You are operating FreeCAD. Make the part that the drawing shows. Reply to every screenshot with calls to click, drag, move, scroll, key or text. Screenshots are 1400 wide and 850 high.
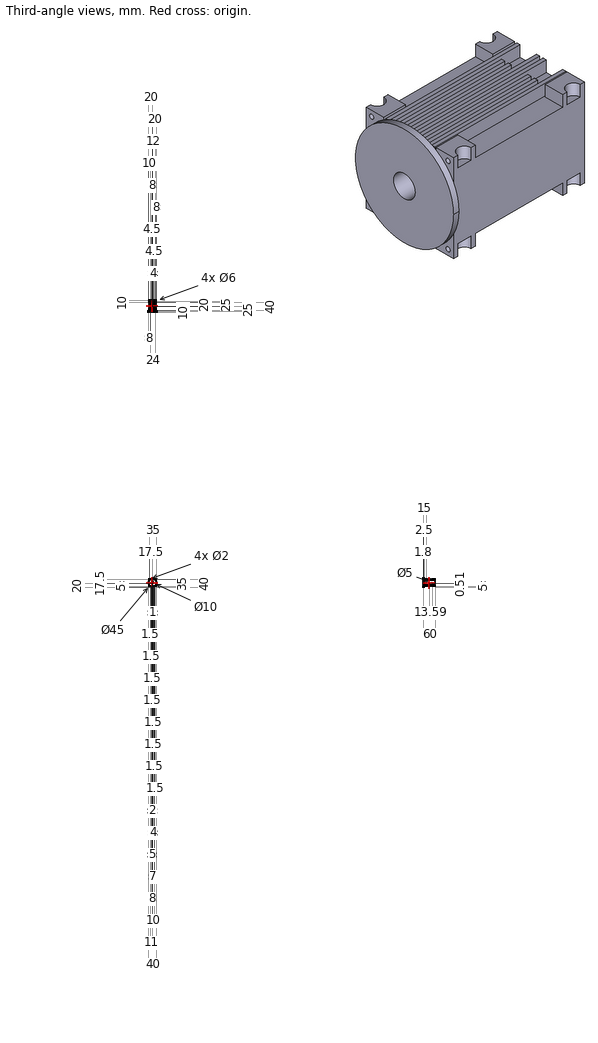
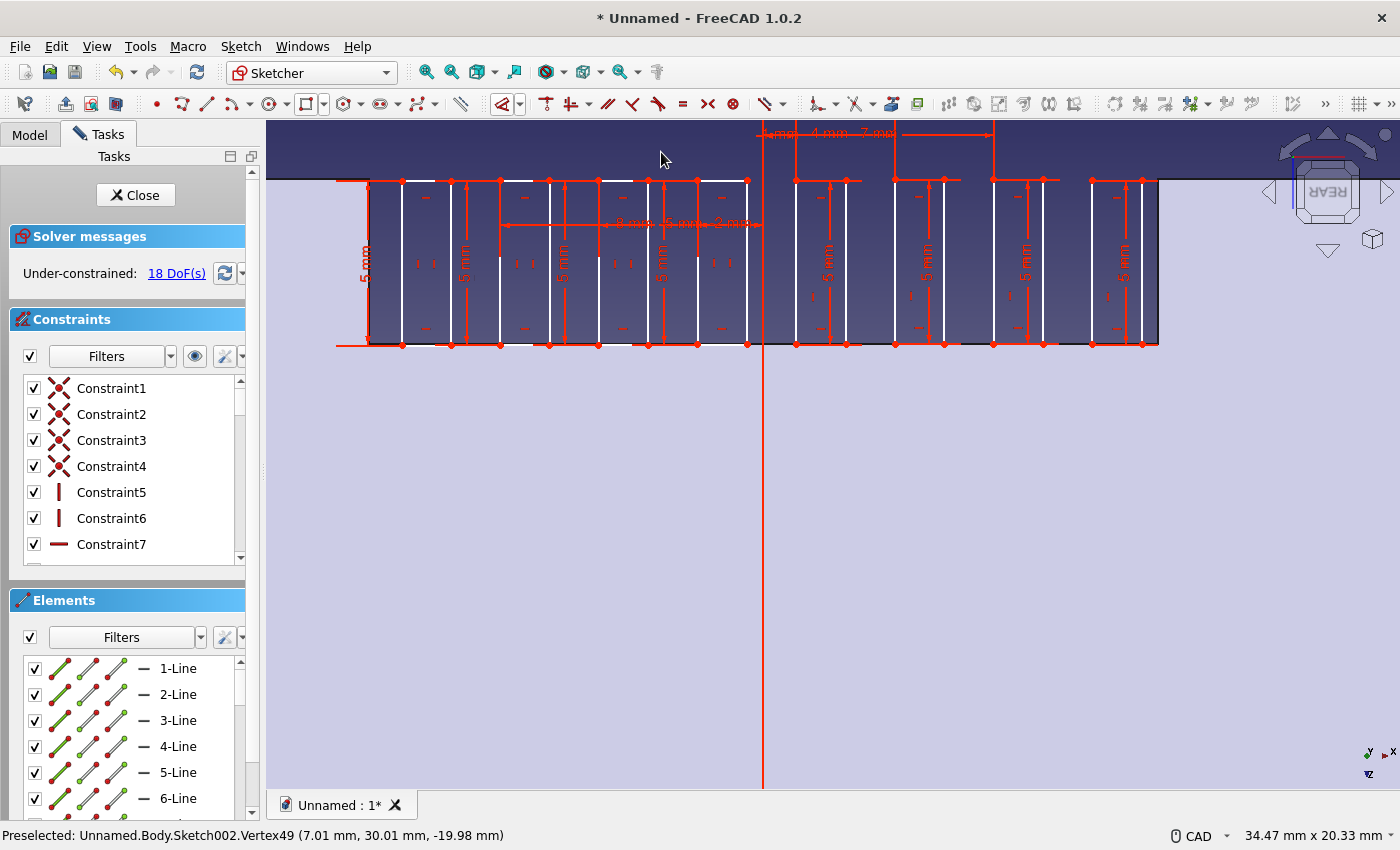
click(417, 346)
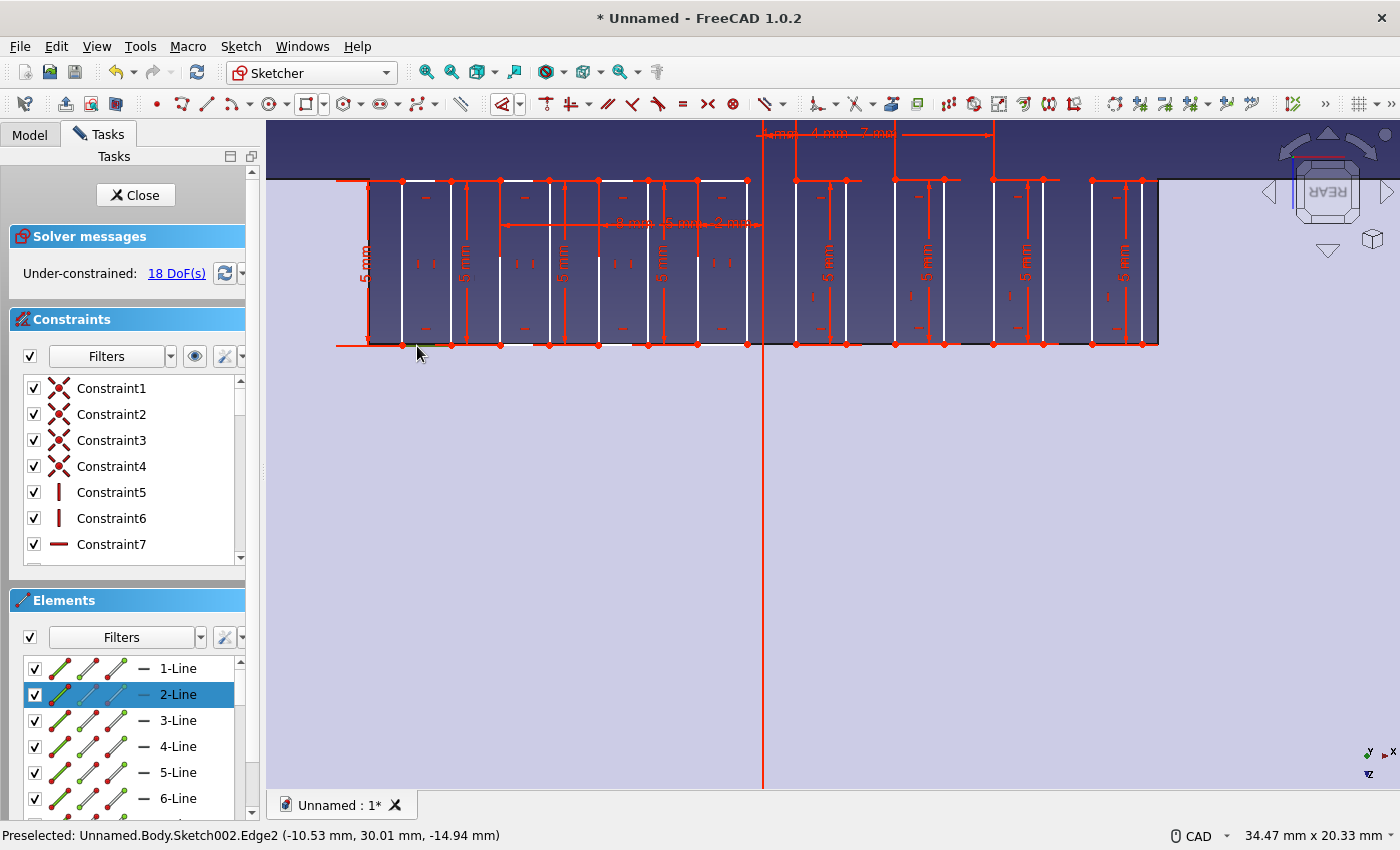
click(520, 104)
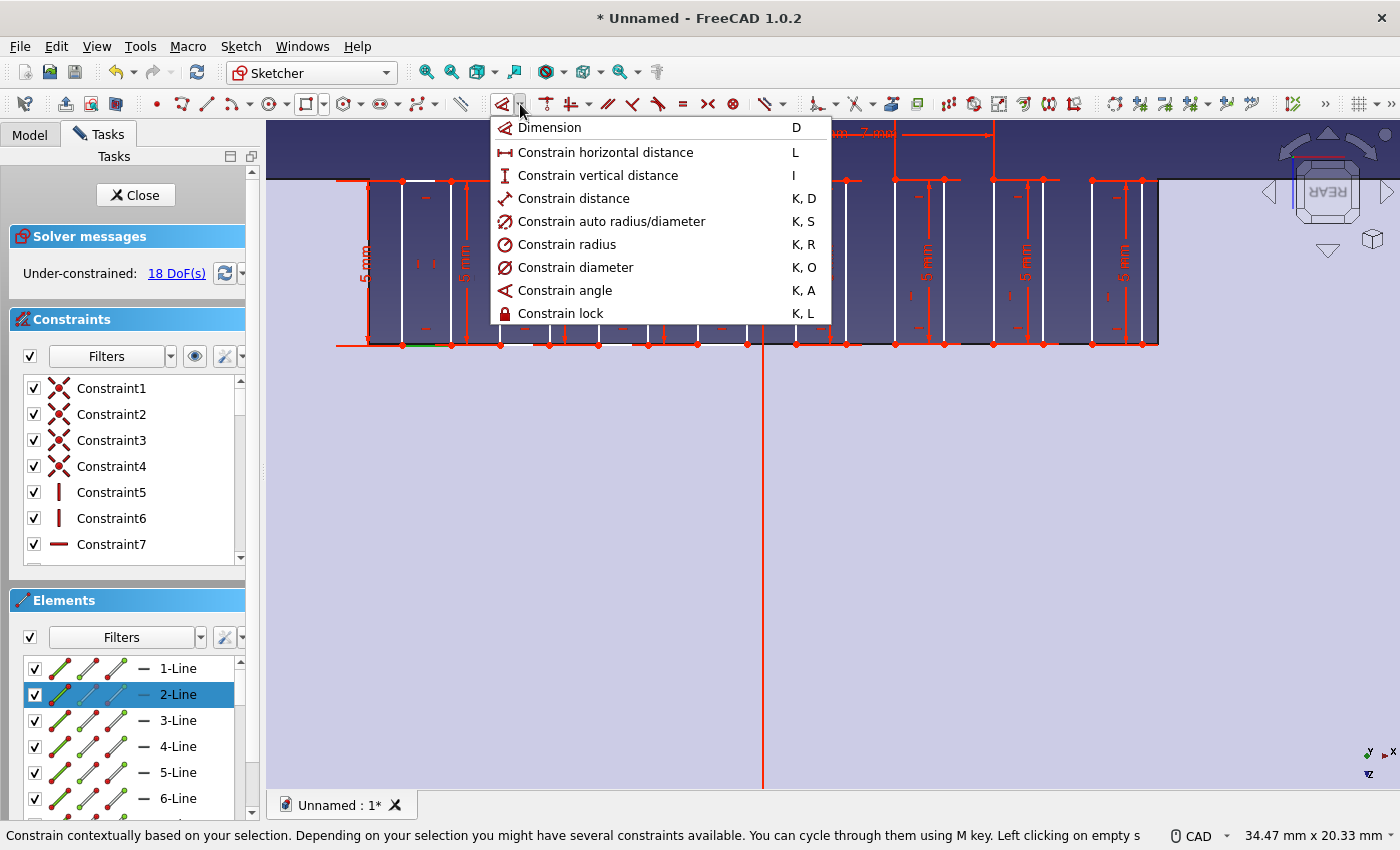
click(661, 152)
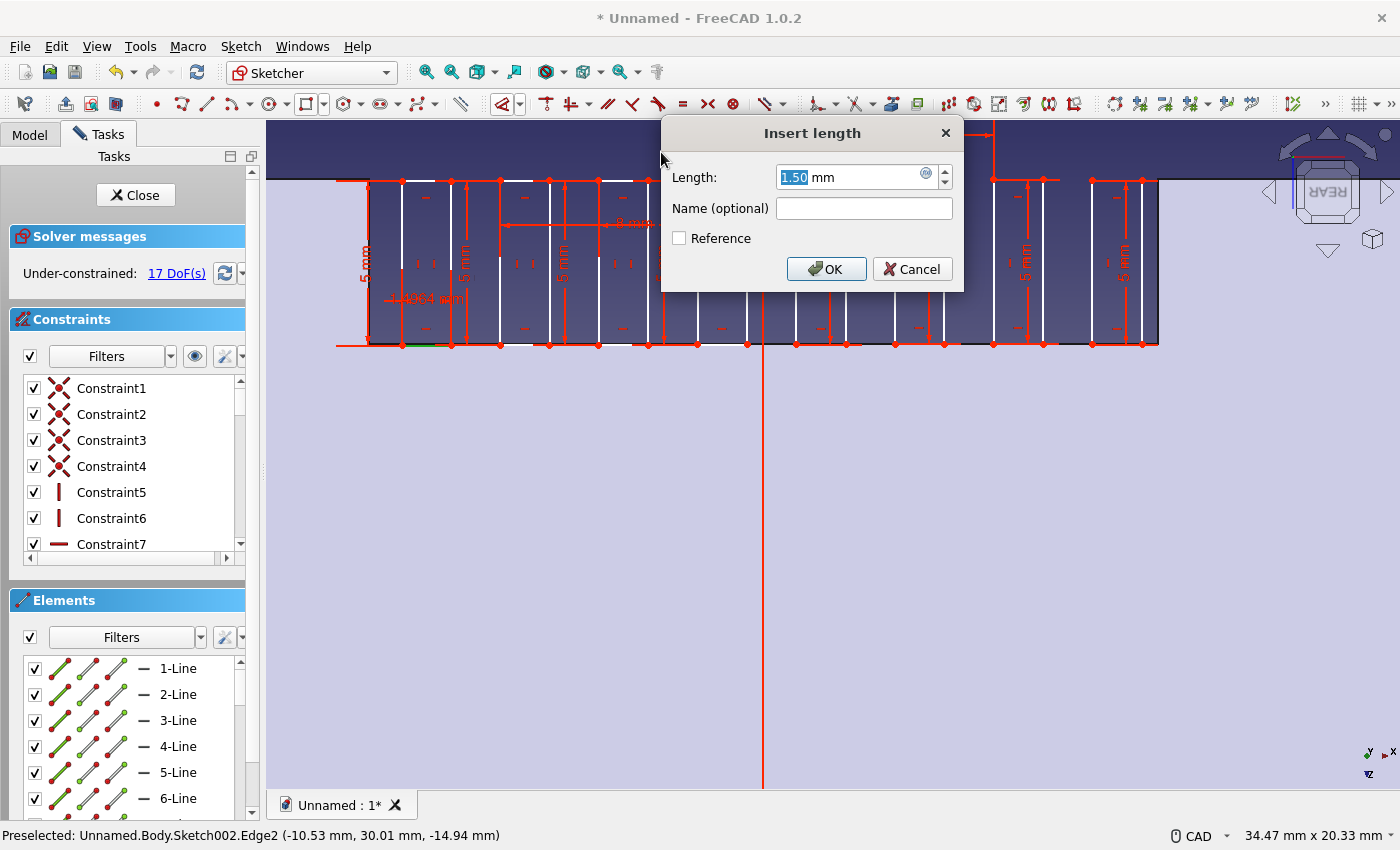
text(1.5)
key(Return)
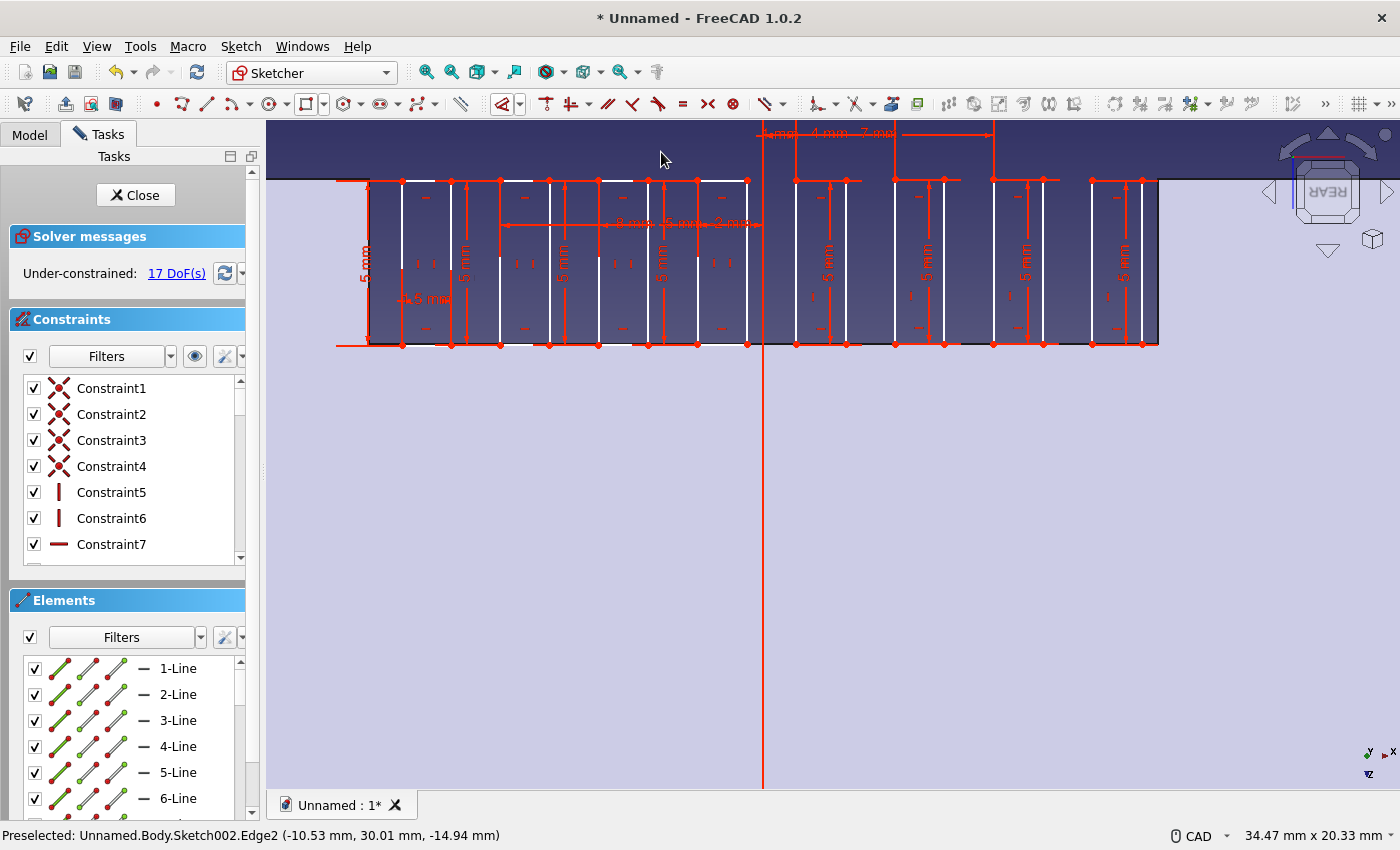
click(515, 345)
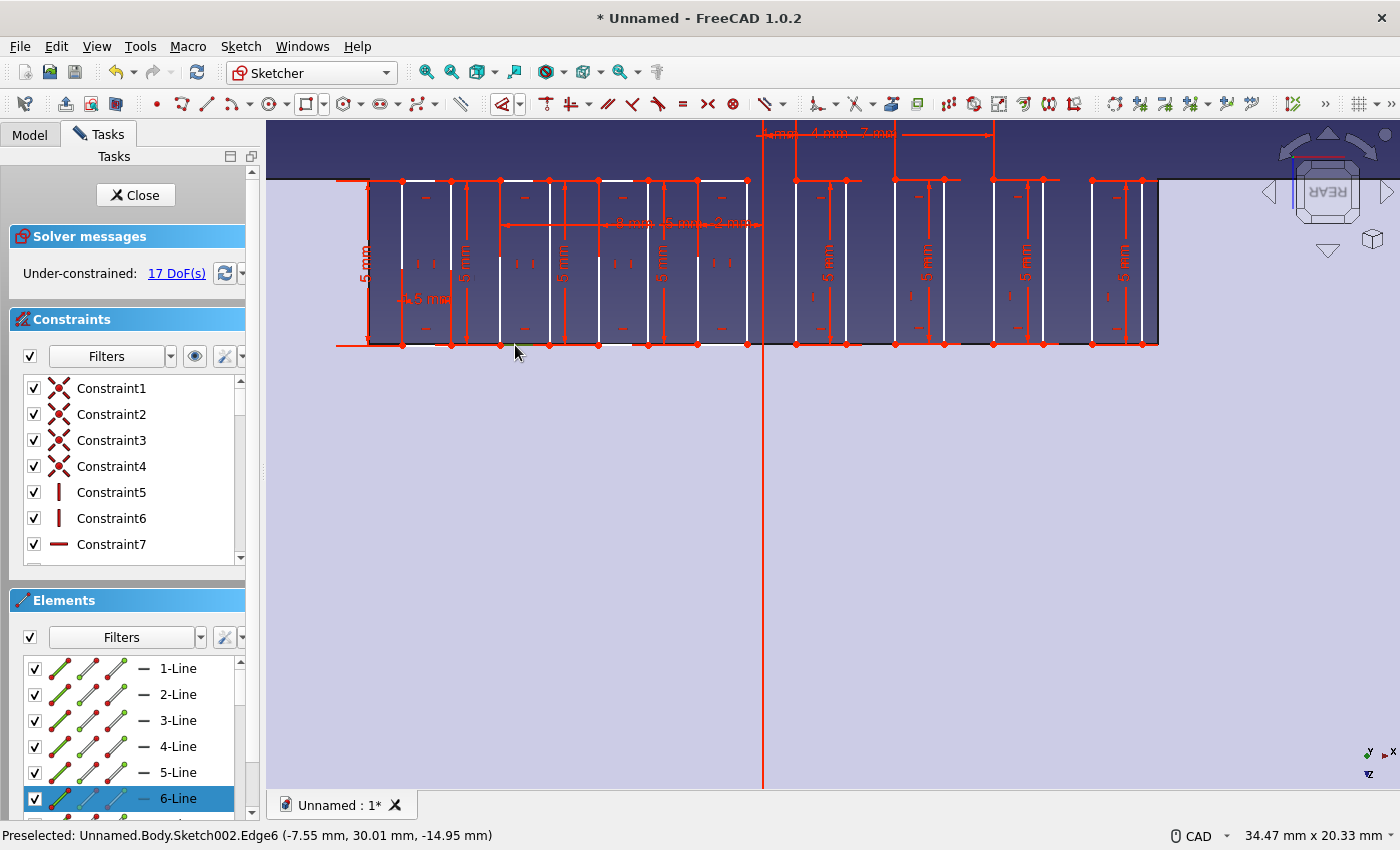
key(l)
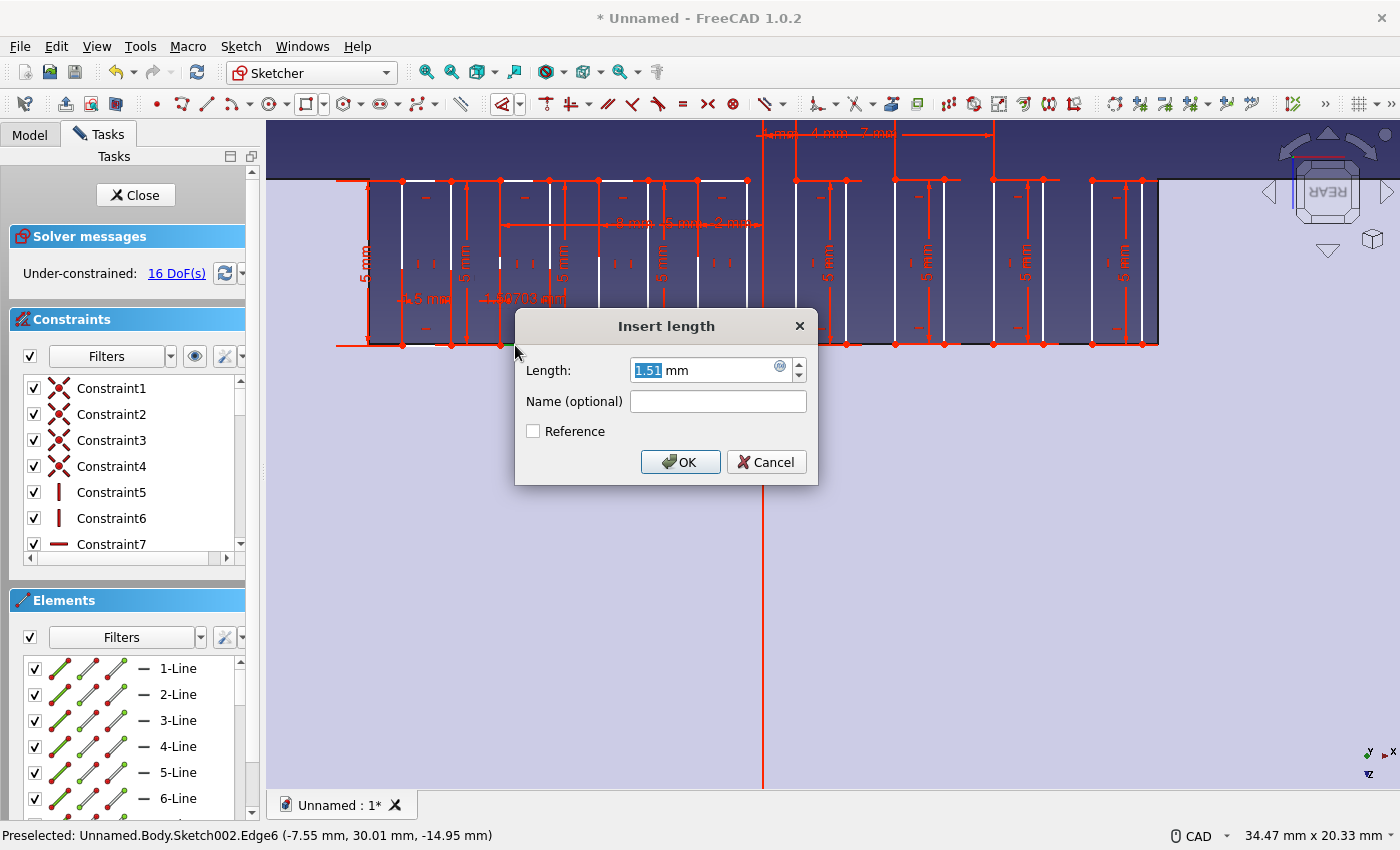
text(1.5)
key(Return)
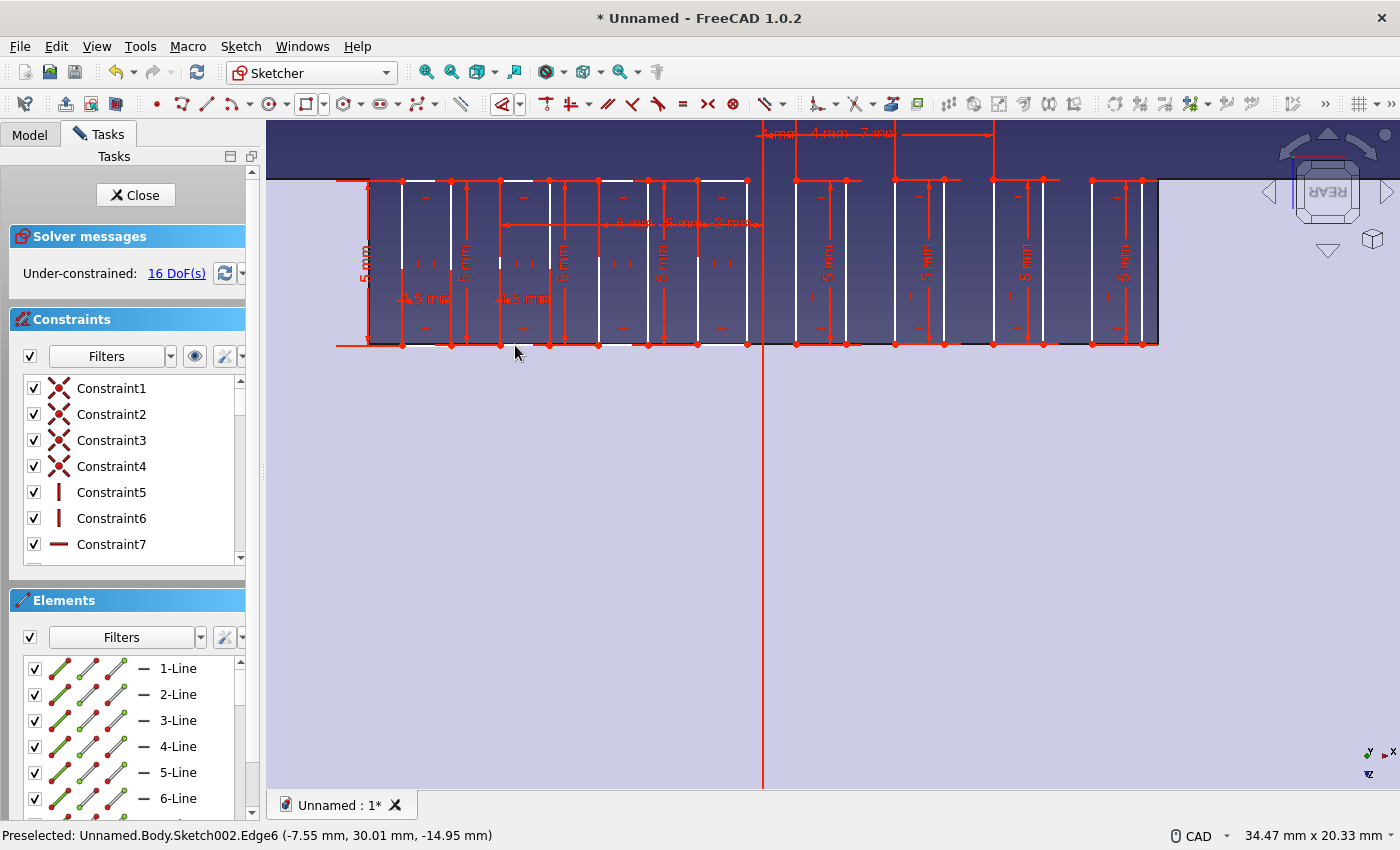
click(614, 345)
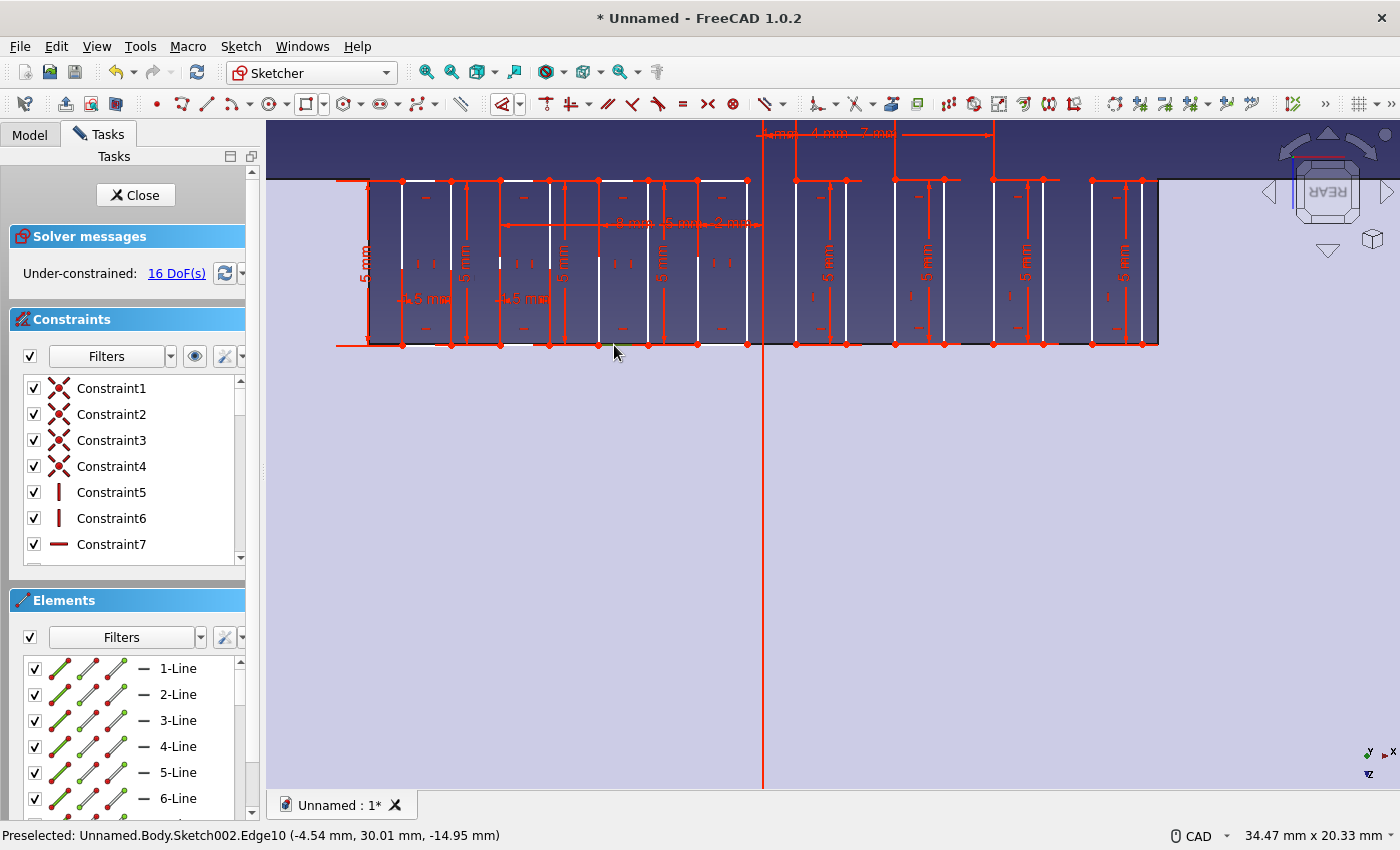
click(520, 104)